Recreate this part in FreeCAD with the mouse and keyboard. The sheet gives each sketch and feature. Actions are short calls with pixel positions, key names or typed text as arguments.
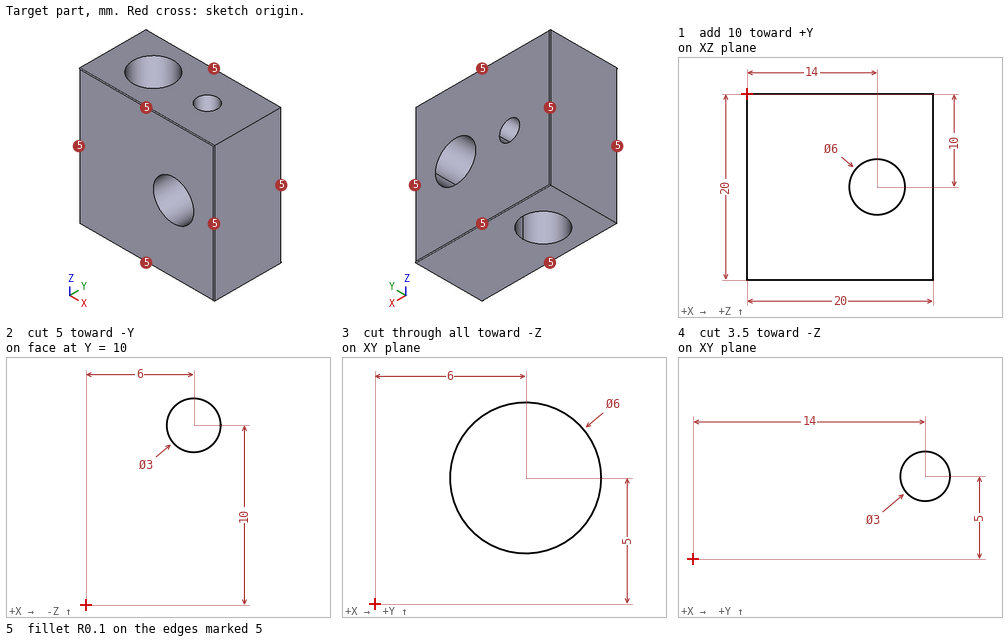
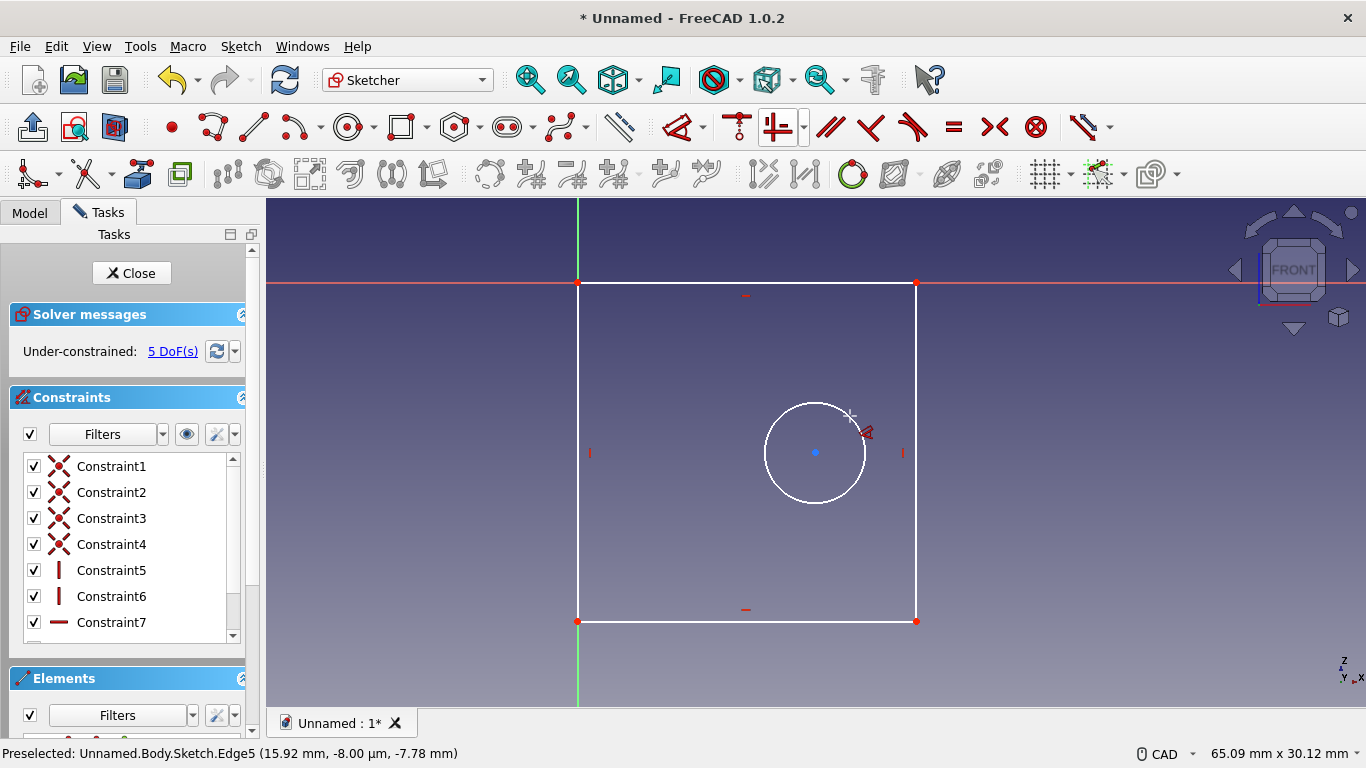
click(850, 417)
click(872, 394)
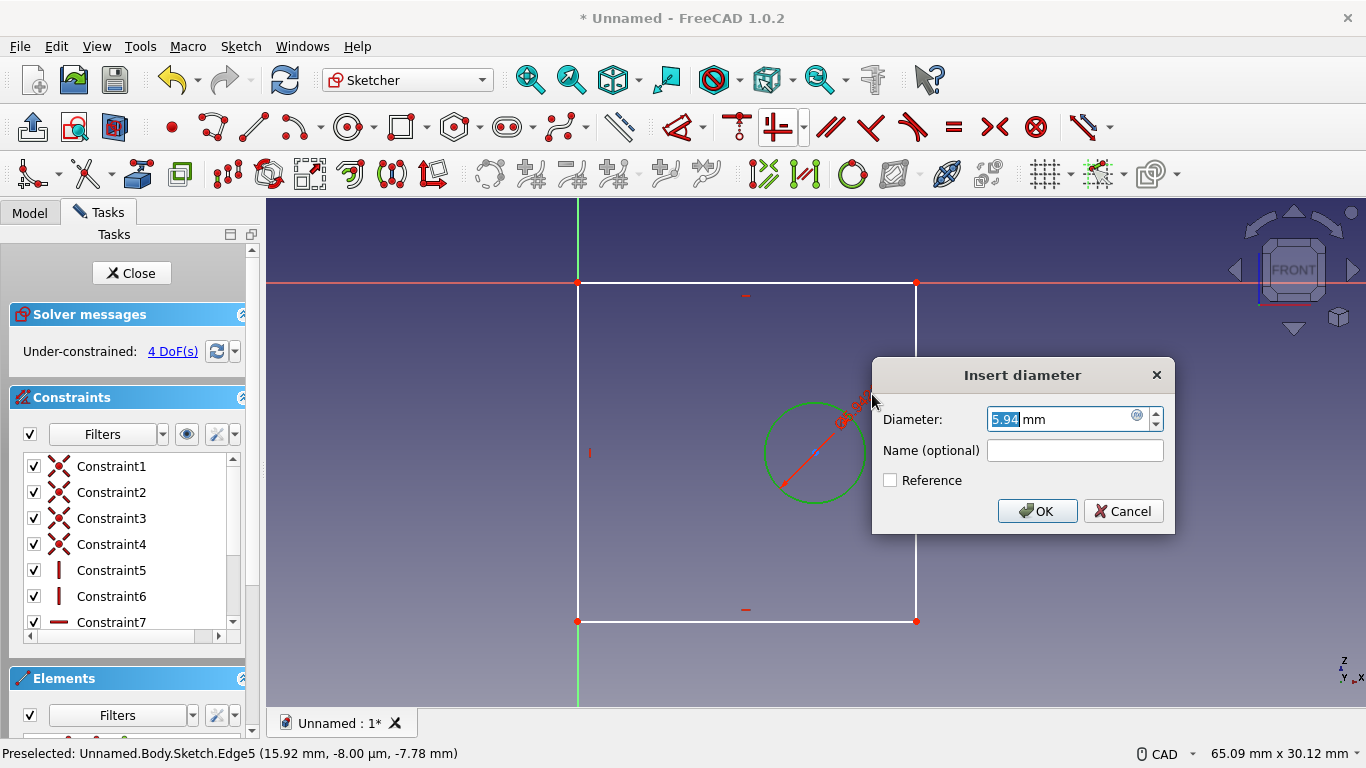
text(6)
key(Return)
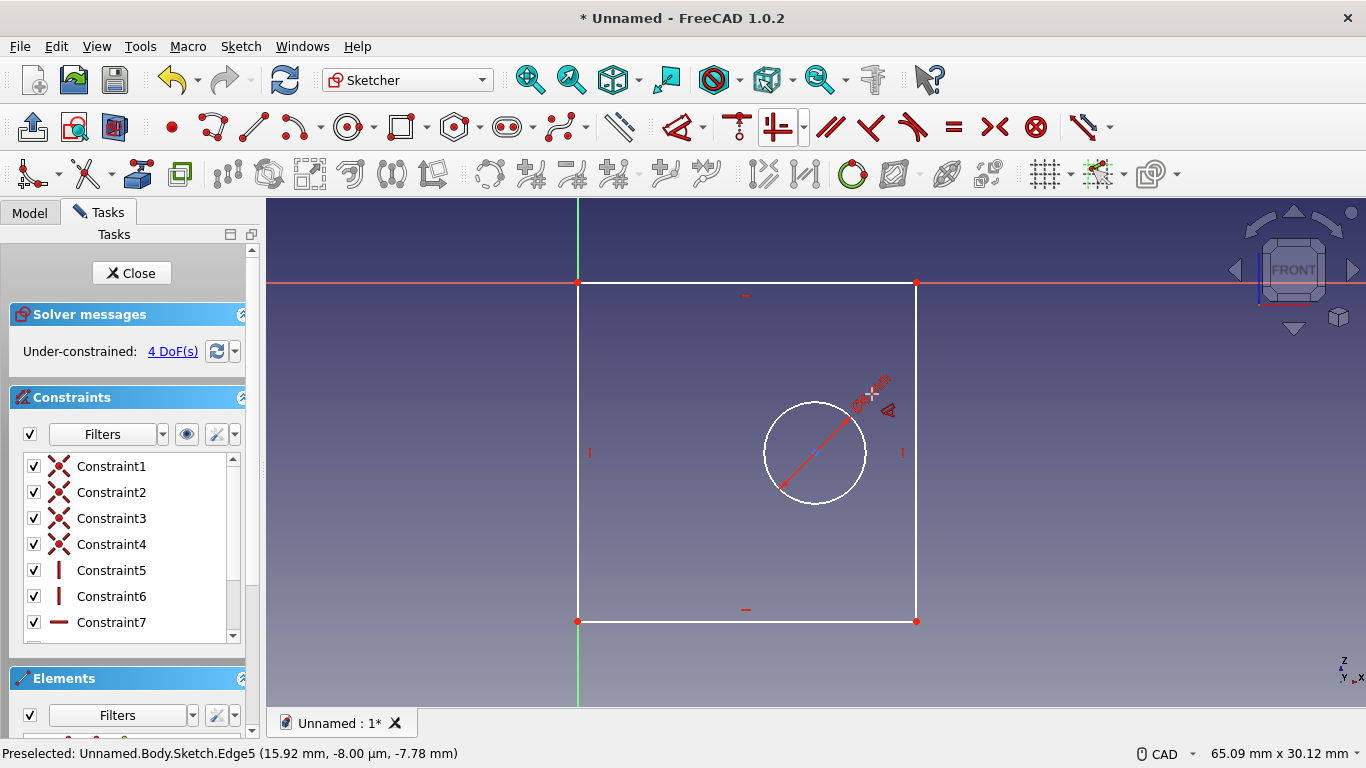
click(578, 385)
click(544, 452)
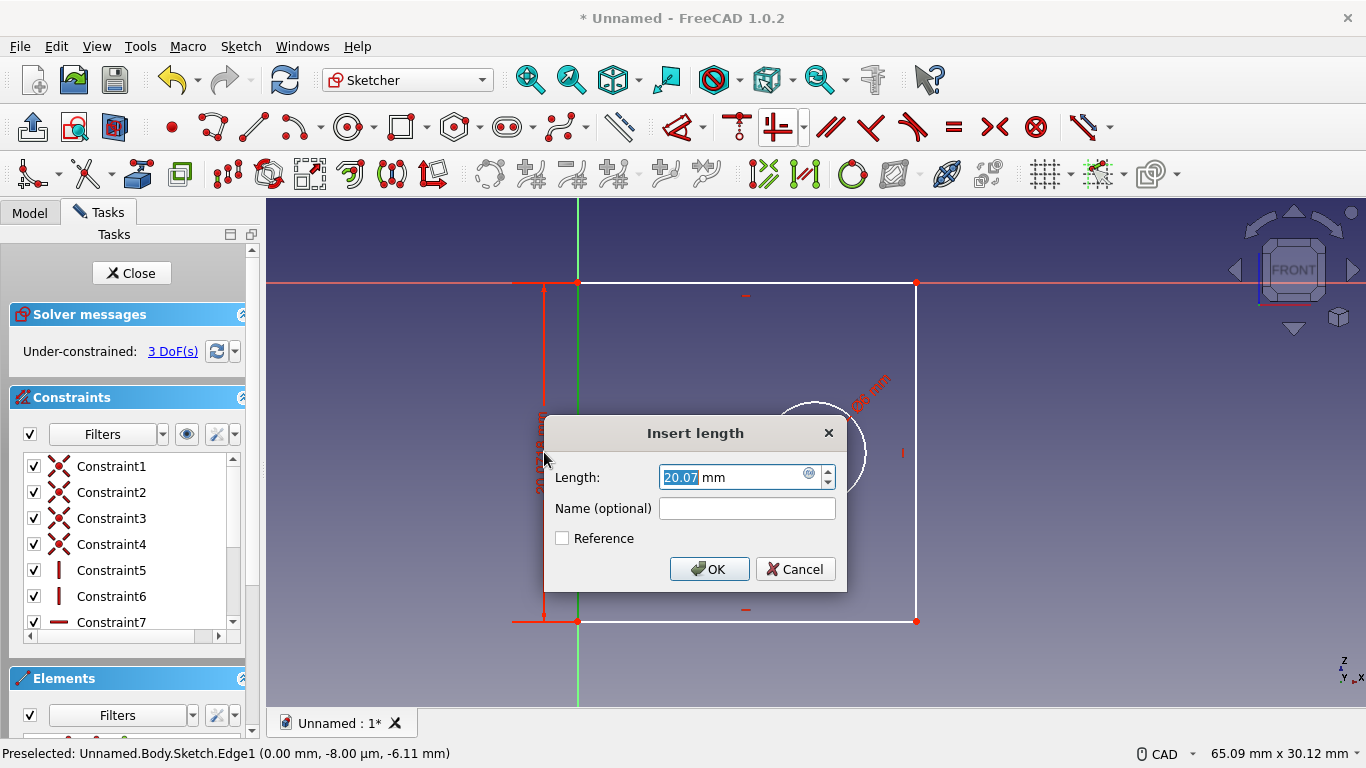
text(20)
key(Return)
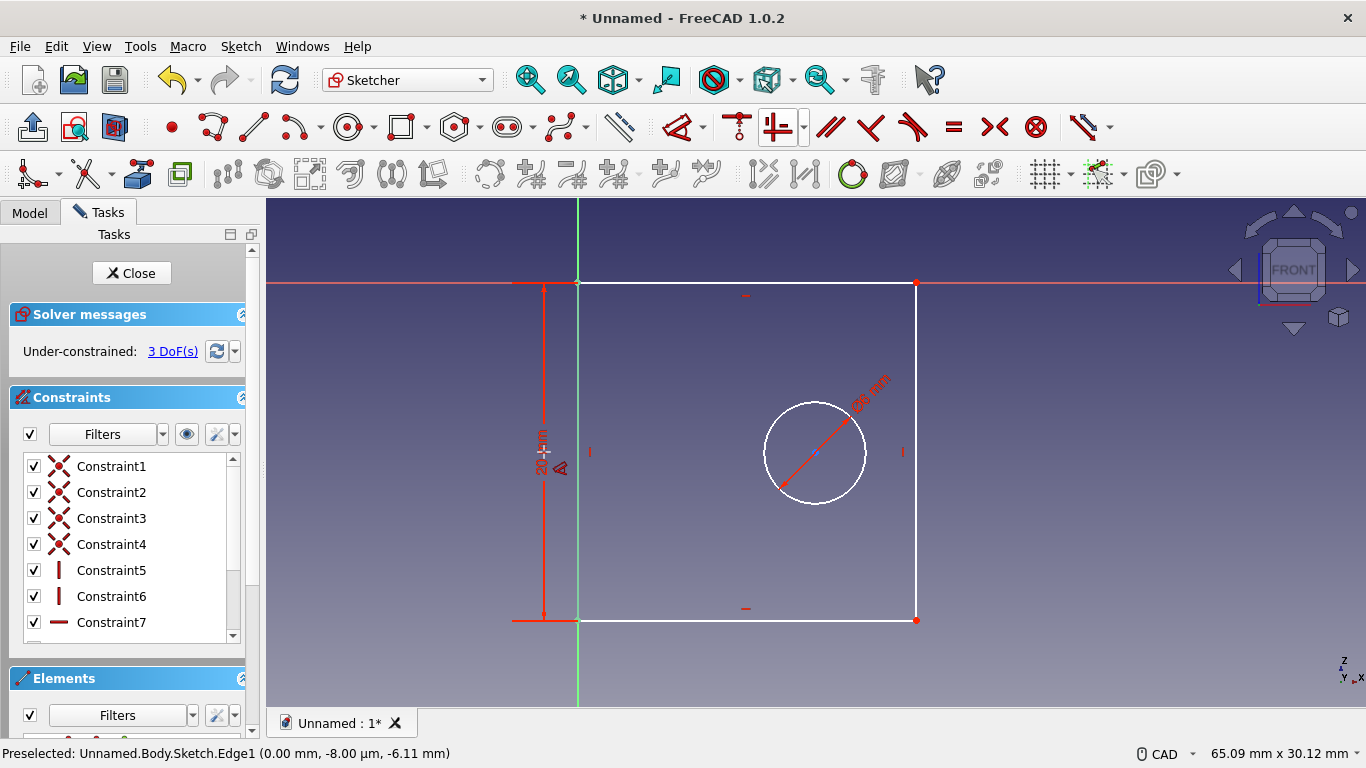
click(679, 621)
click(747, 655)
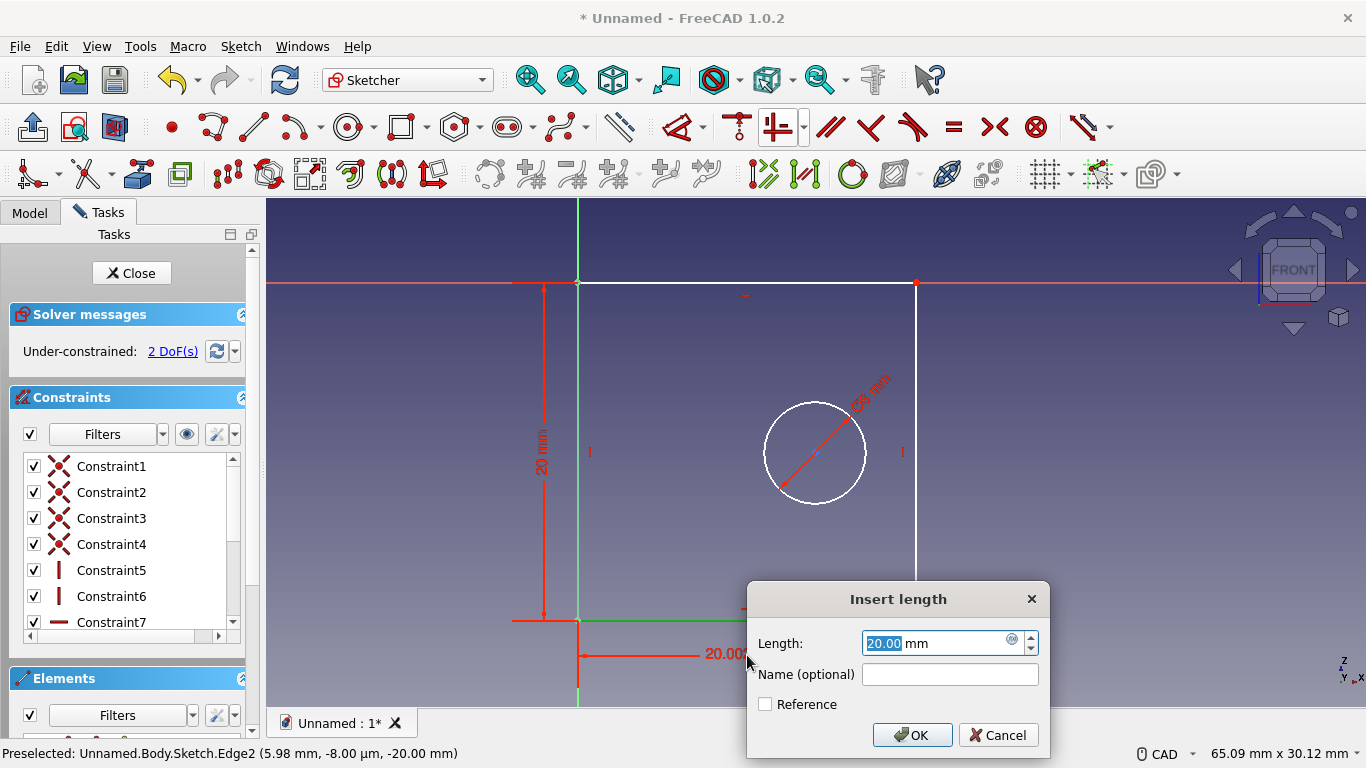
text(20)
key(Return)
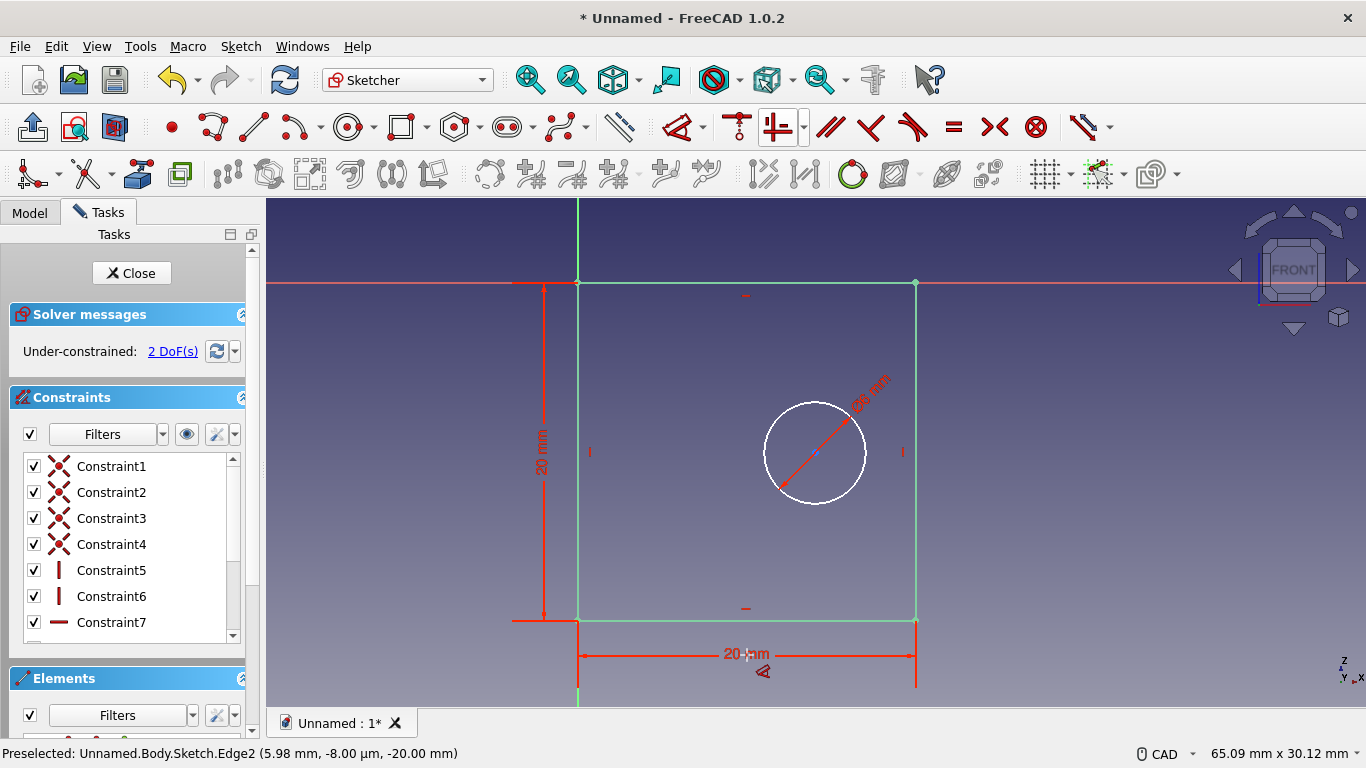
click(815, 453)
click(696, 249)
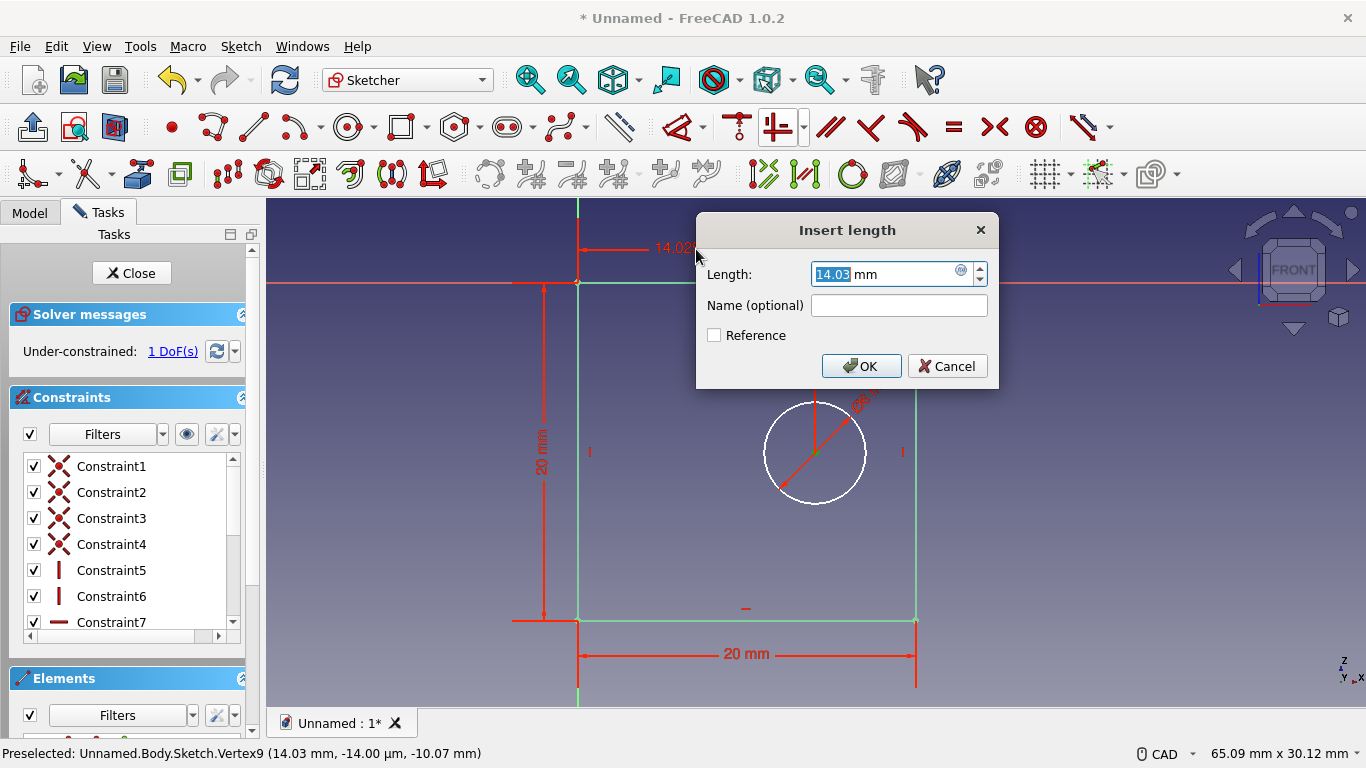
text(14)
key(Return)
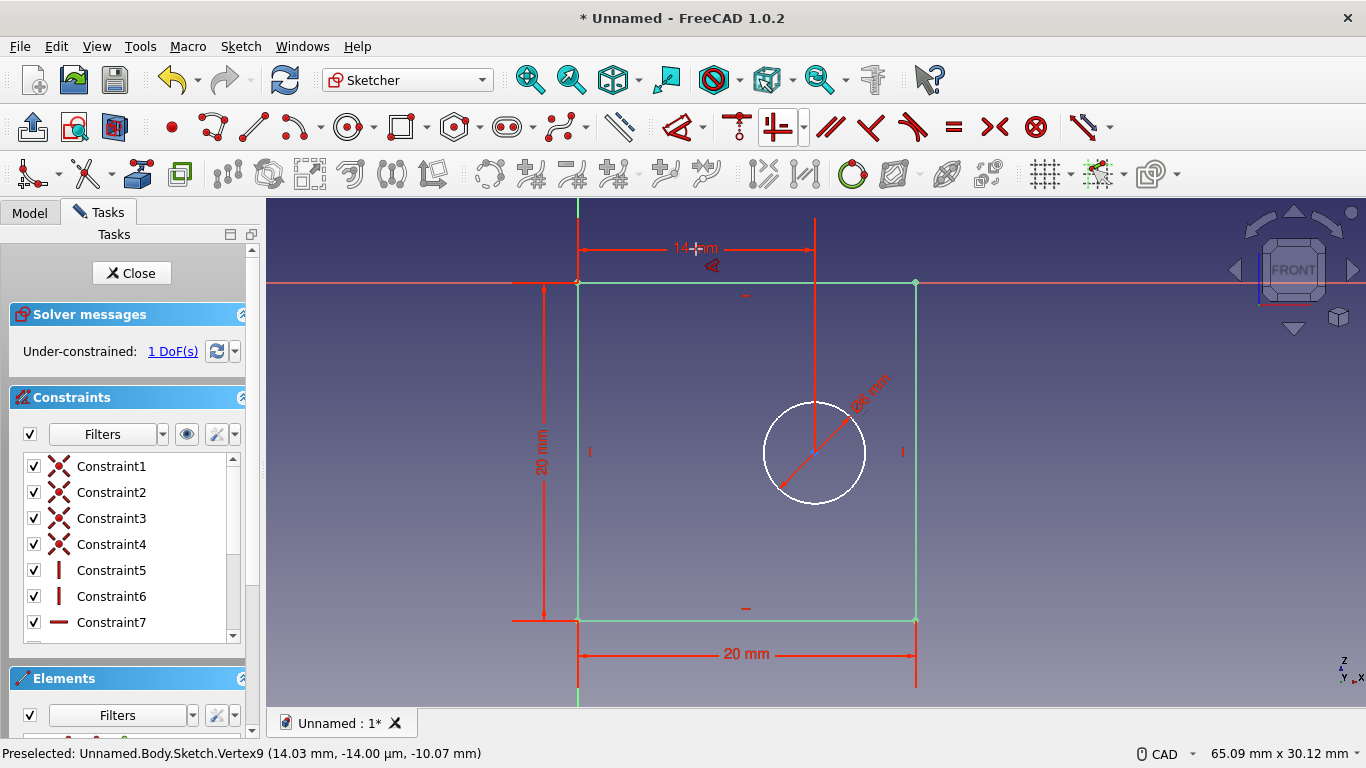
click(815, 453)
click(544, 368)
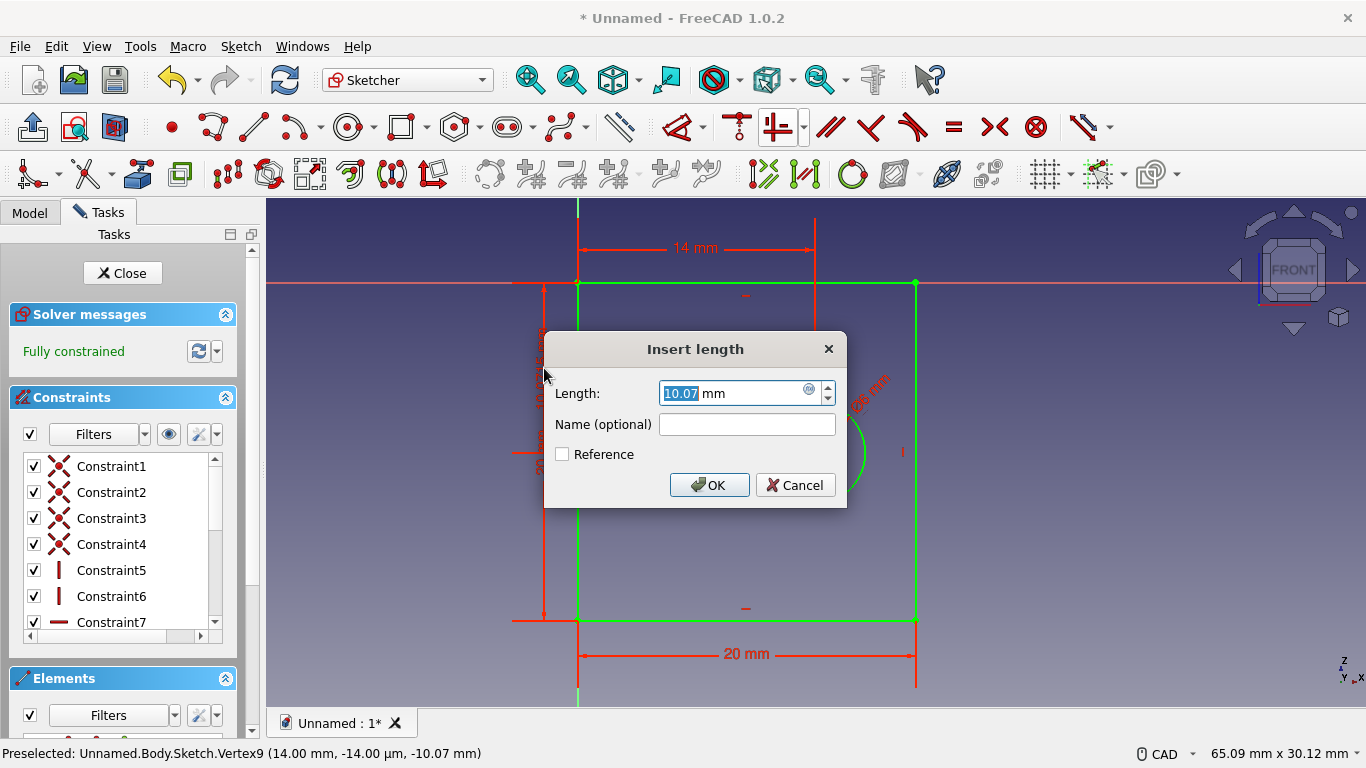
text(10)
key(Return)
key(Escape)